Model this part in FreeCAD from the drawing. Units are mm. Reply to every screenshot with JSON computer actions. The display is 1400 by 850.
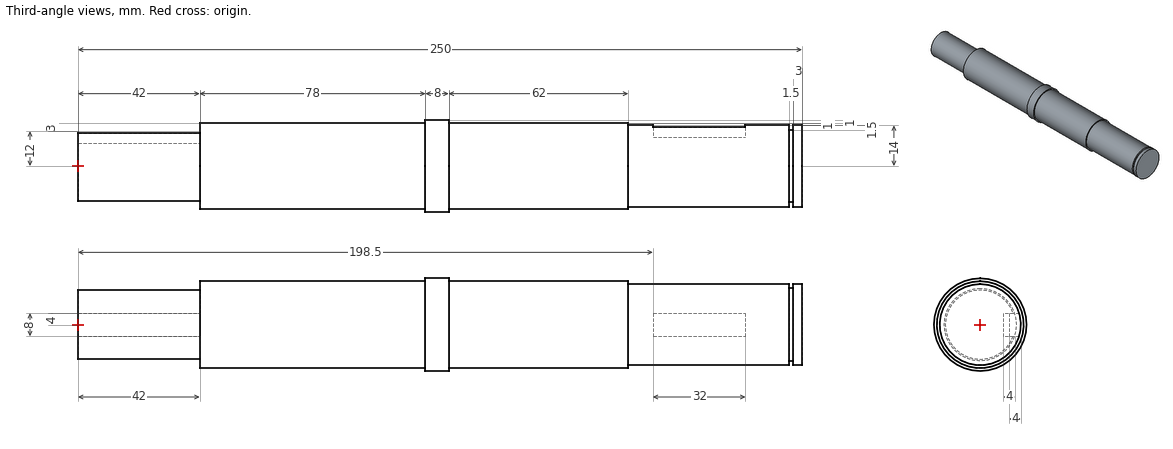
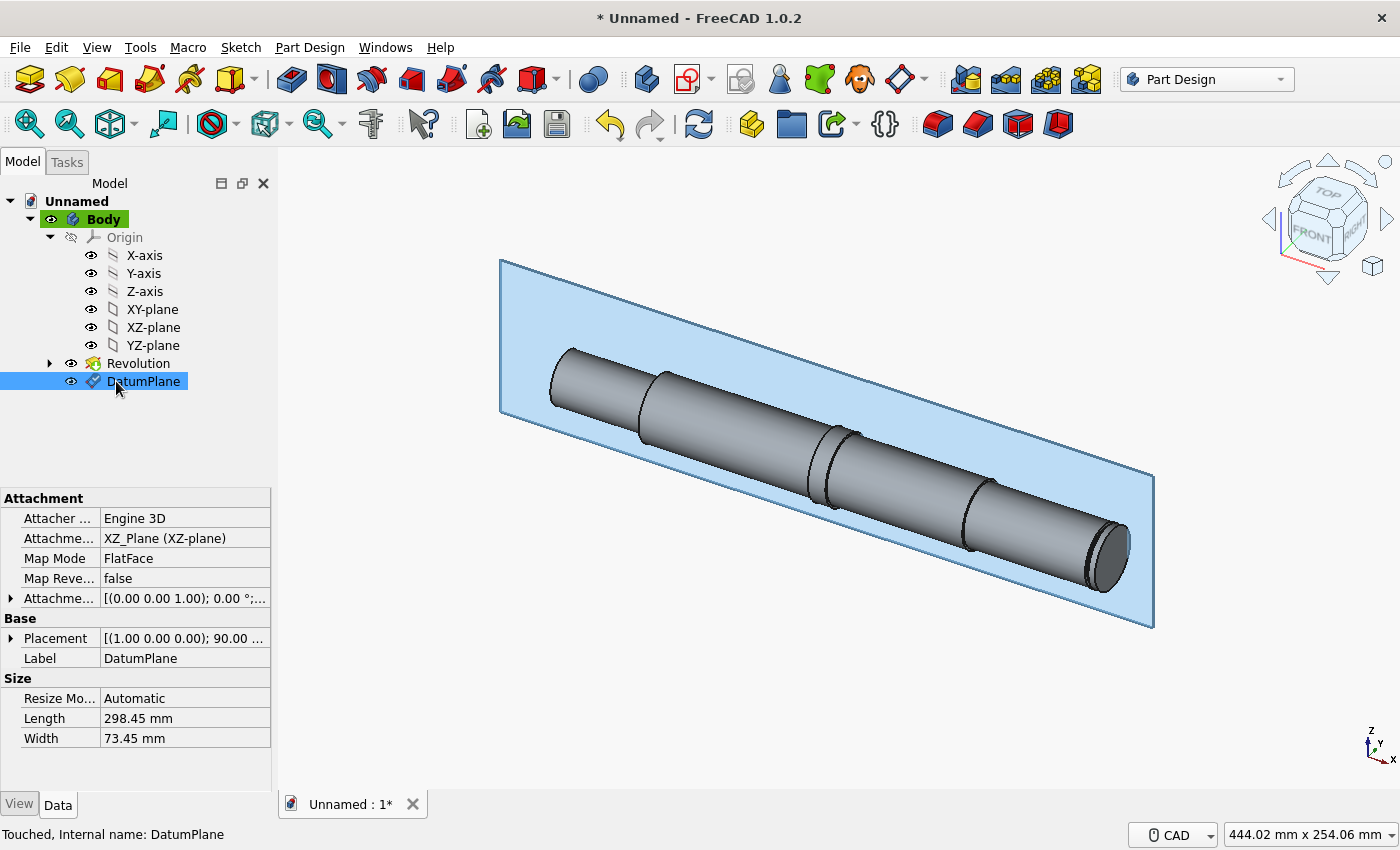
{"action": "left_click", "coordinate": [688, 80]}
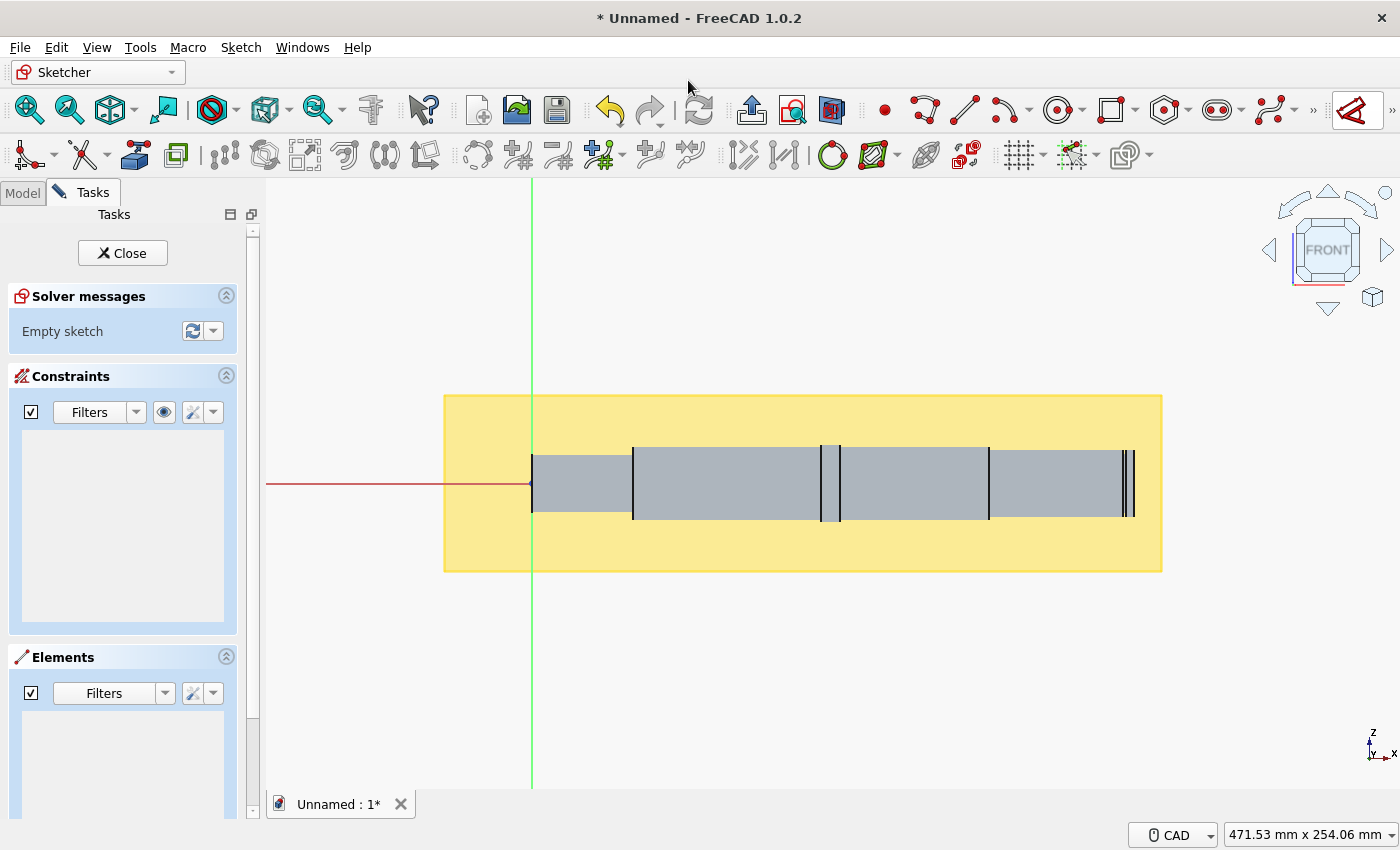
{"action": "left_click", "coordinate": [832, 110]}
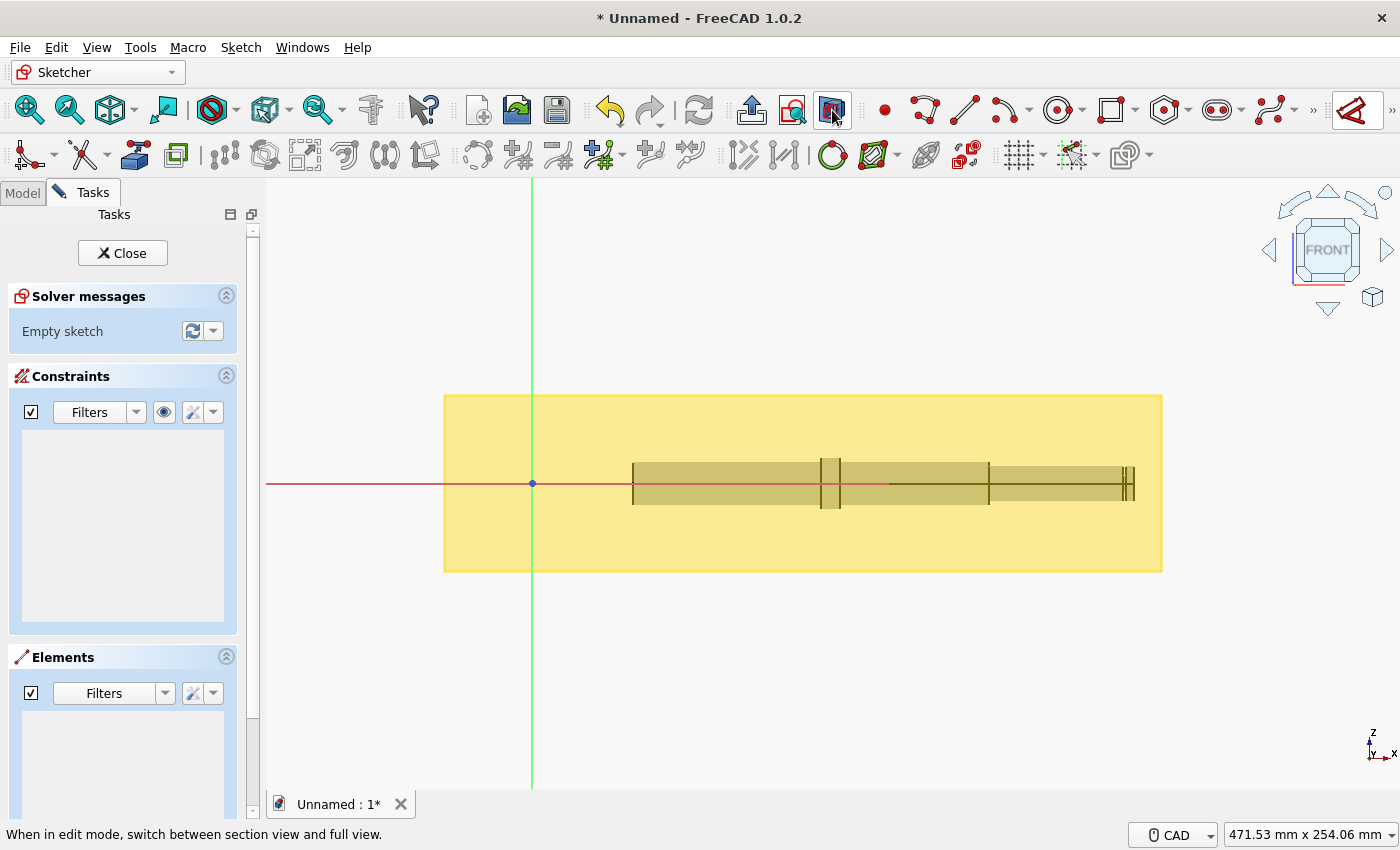
{"action": "scroll", "coordinate": [547, 484], "scroll_direction": "up", "scroll_amount": 9}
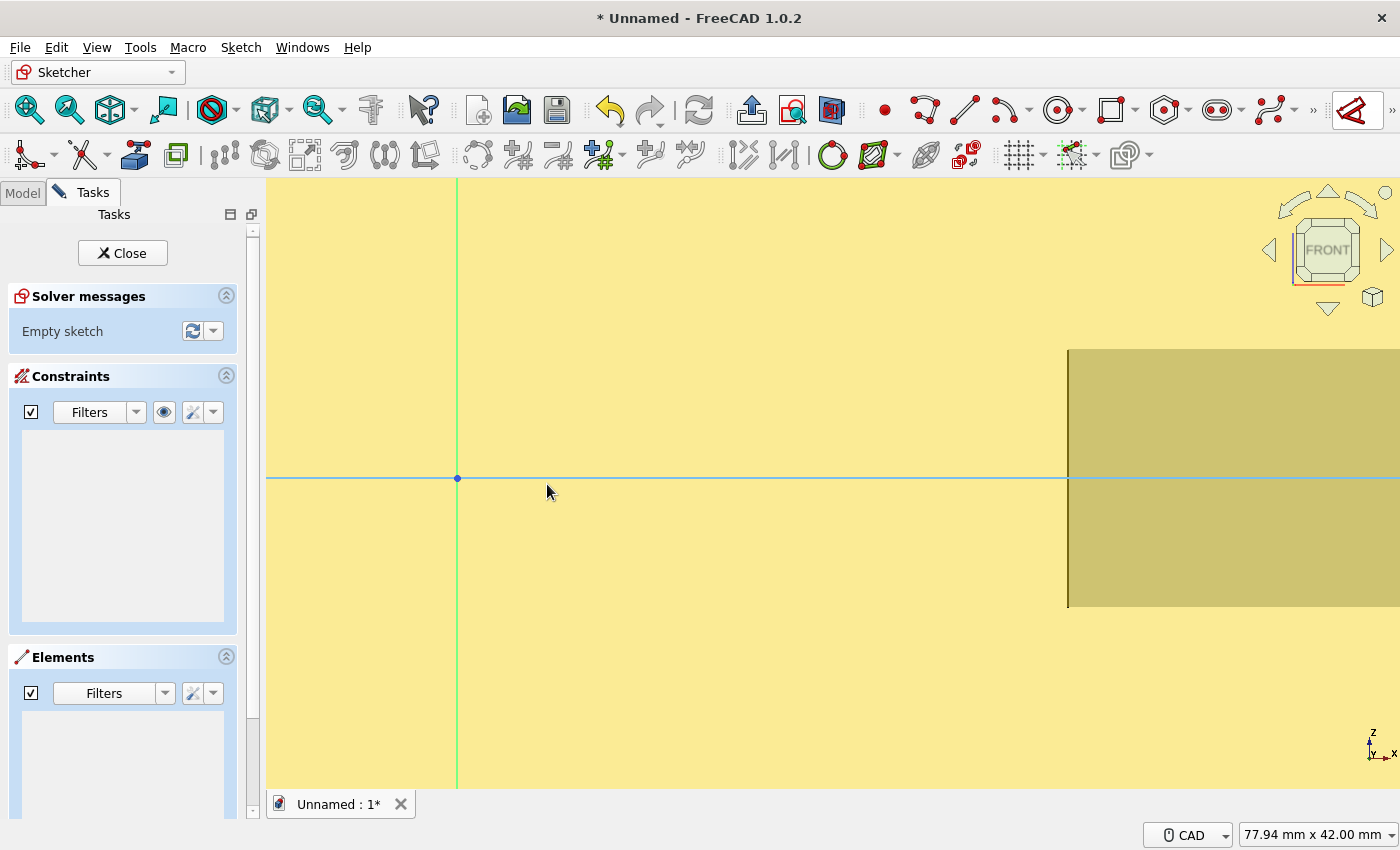
{"action": "left_click", "coordinate": [1112, 110]}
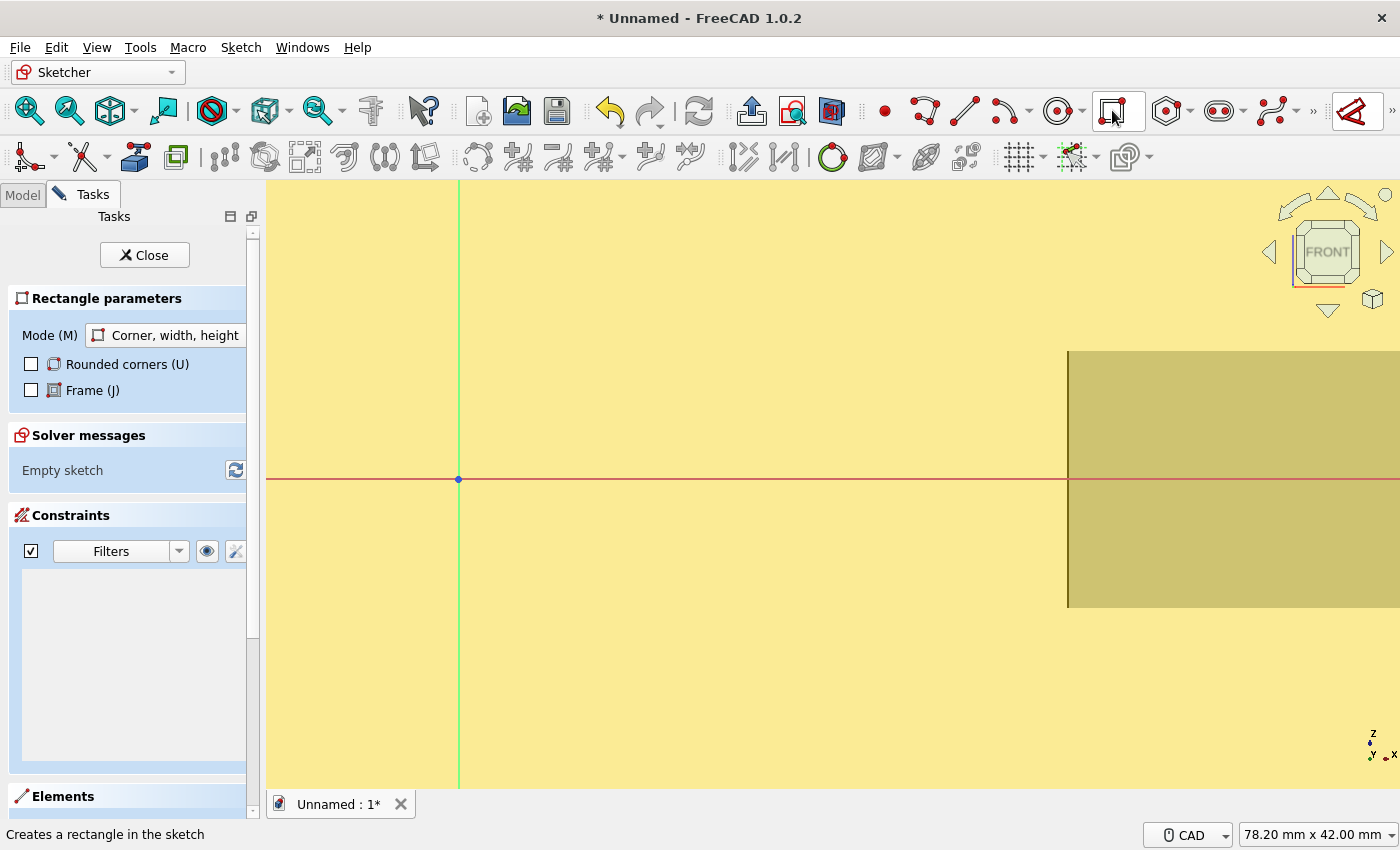
{"action": "left_click", "coordinate": [459, 421]}
{"action": "mouse_move", "coordinate": [1068, 537]}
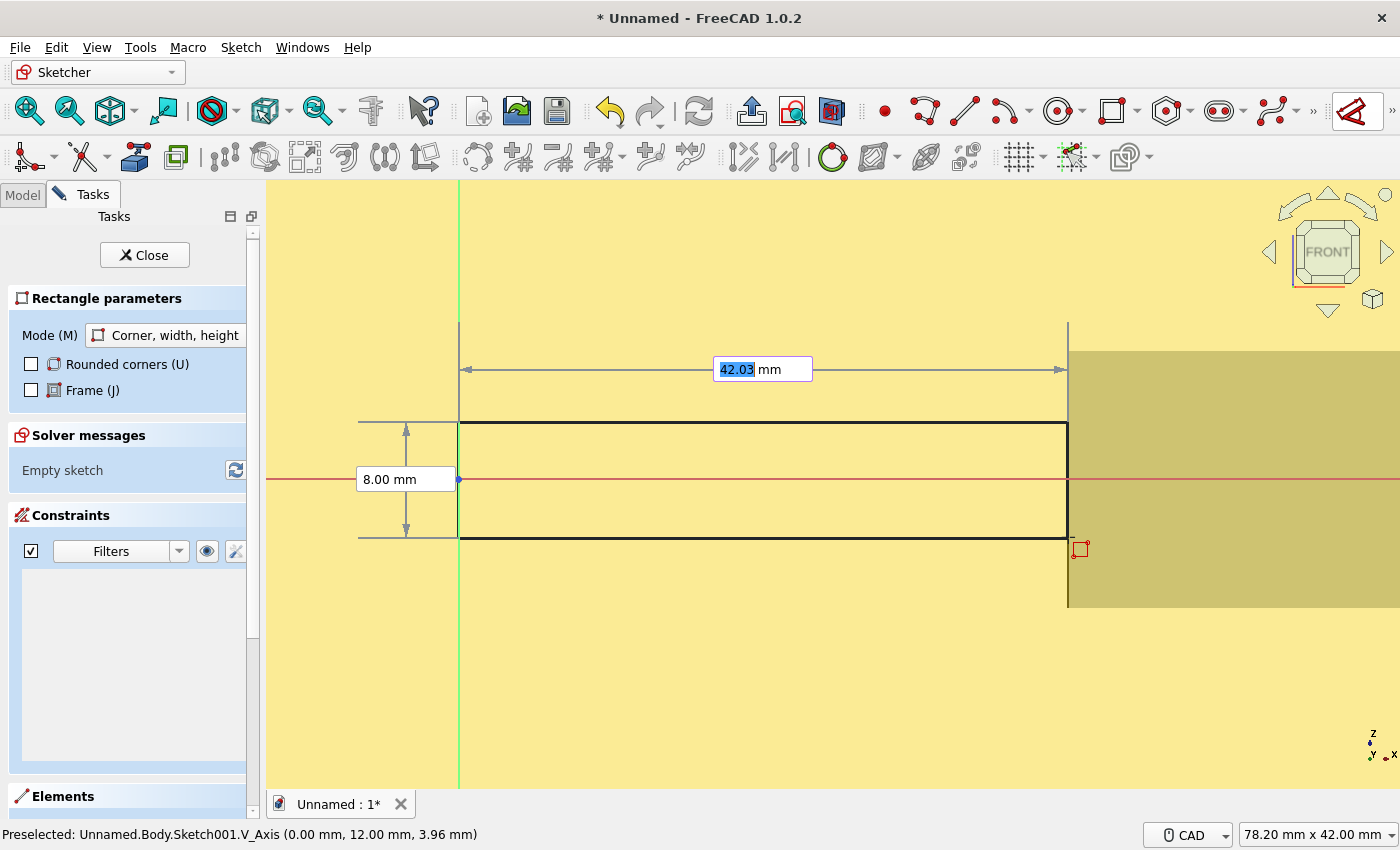
{"action": "type", "text": "42"}
{"action": "key", "text": "Tab"}
{"action": "type", "text": "8"}
{"action": "key", "text": "Return"}
{"action": "key", "text": "Escape"}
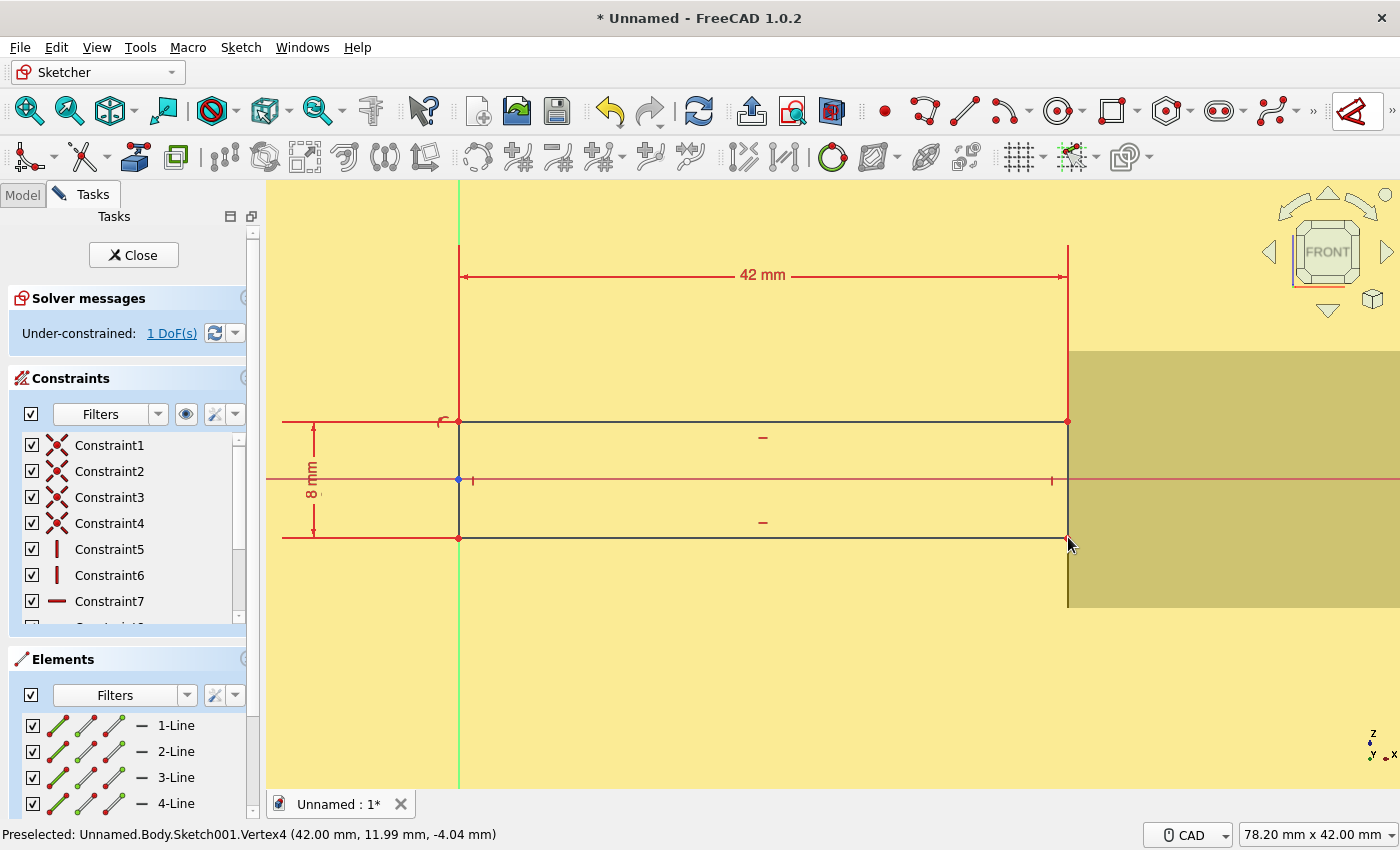
{"action": "left_click", "coordinate": [459, 422]}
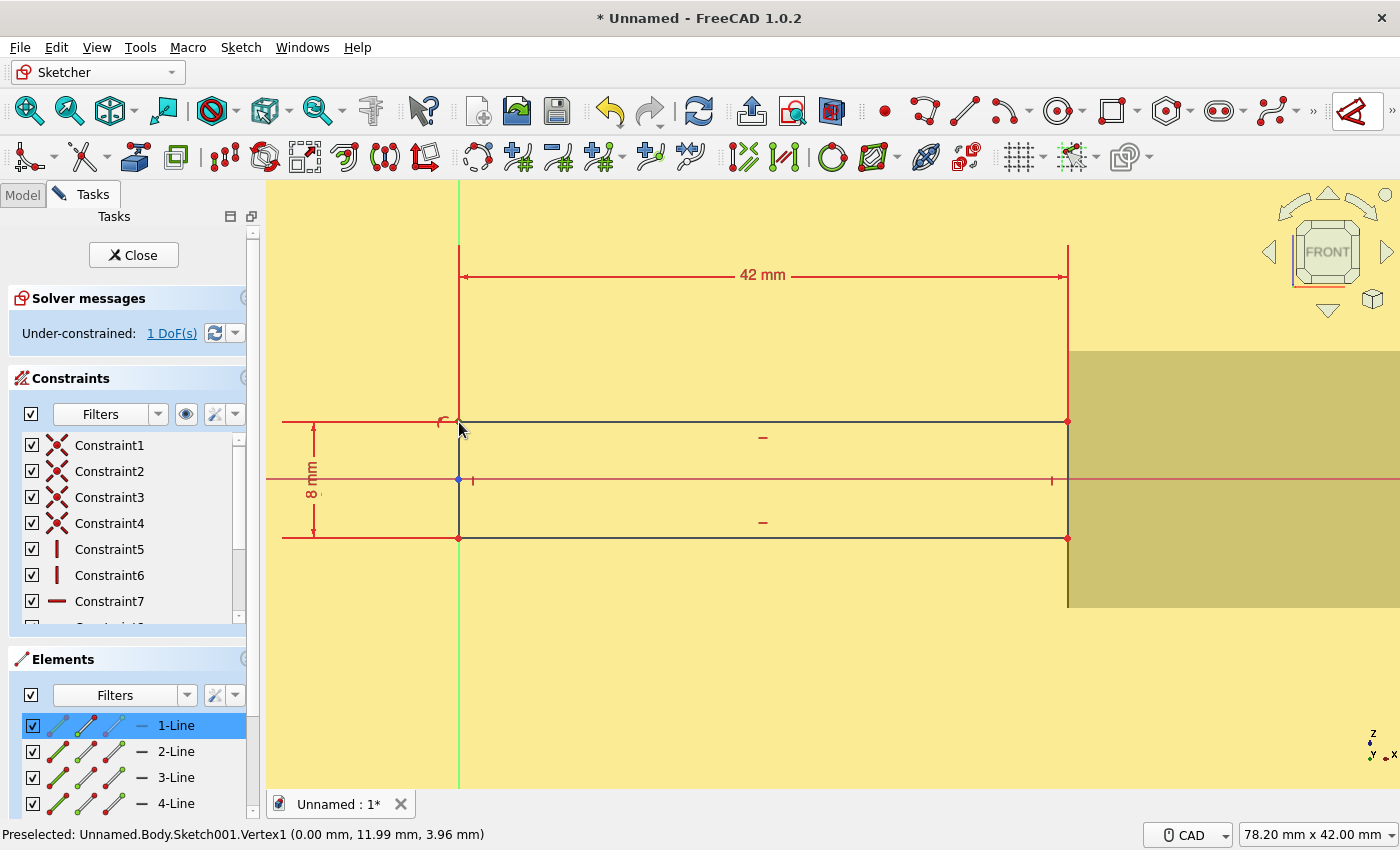
{"action": "left_click", "coordinate": [1378, 112]}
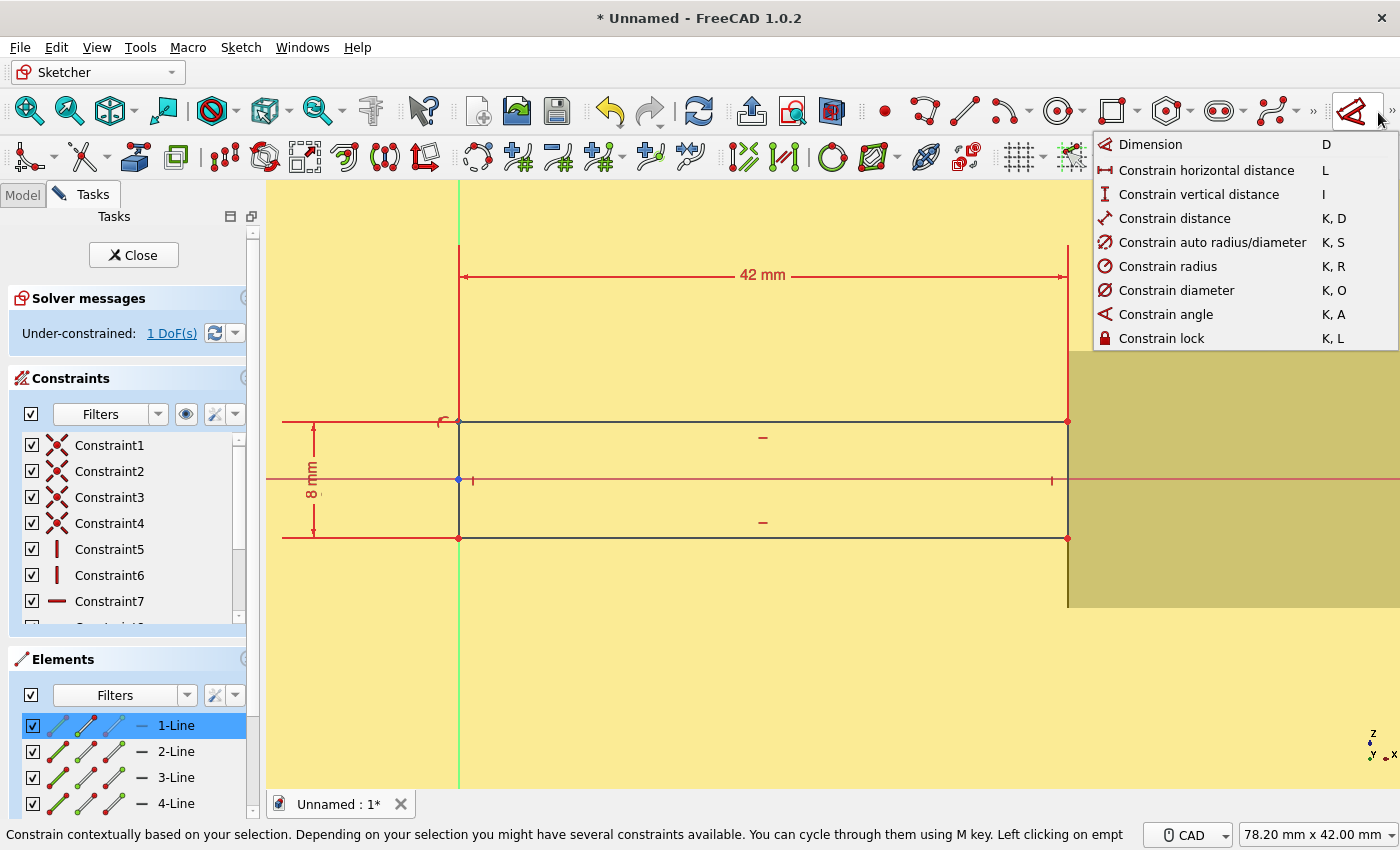
{"action": "left_click", "coordinate": [1246, 194]}